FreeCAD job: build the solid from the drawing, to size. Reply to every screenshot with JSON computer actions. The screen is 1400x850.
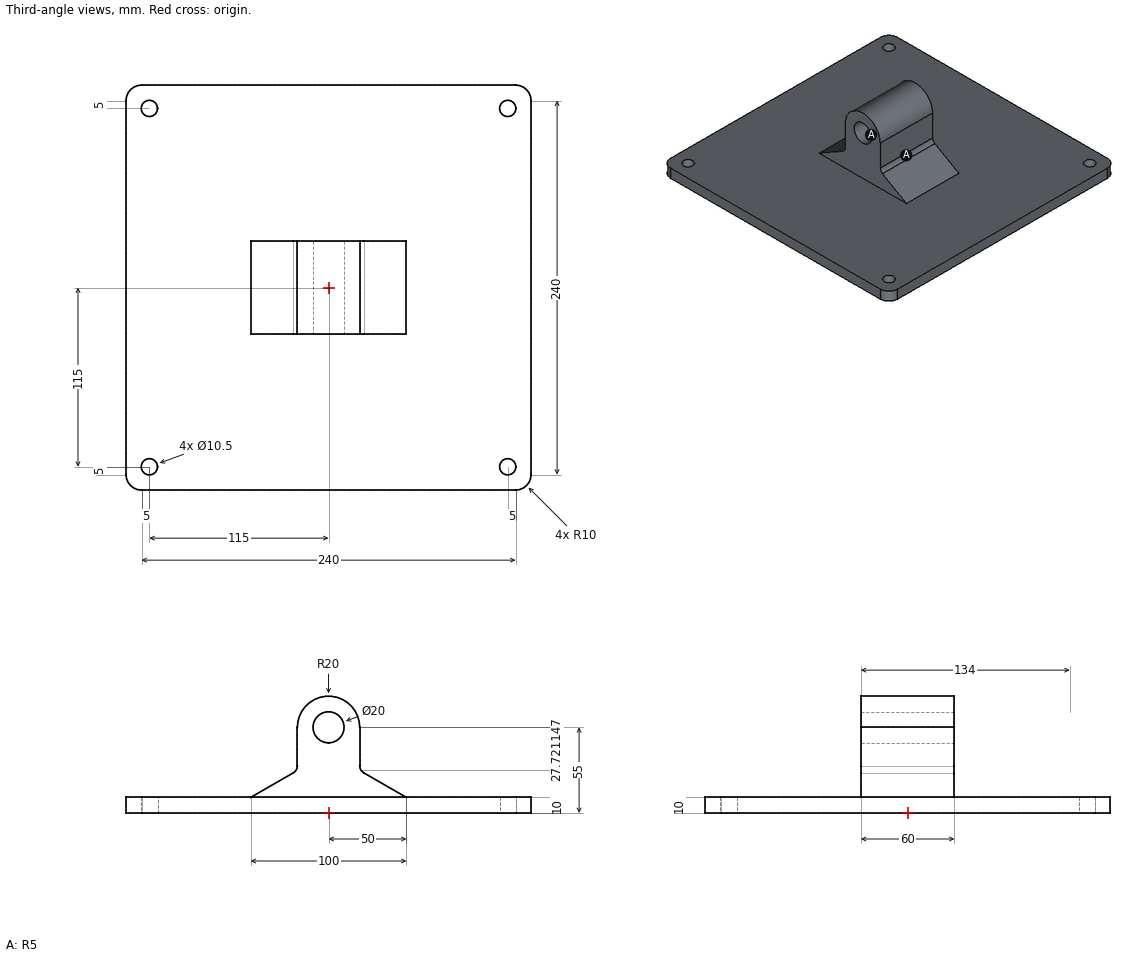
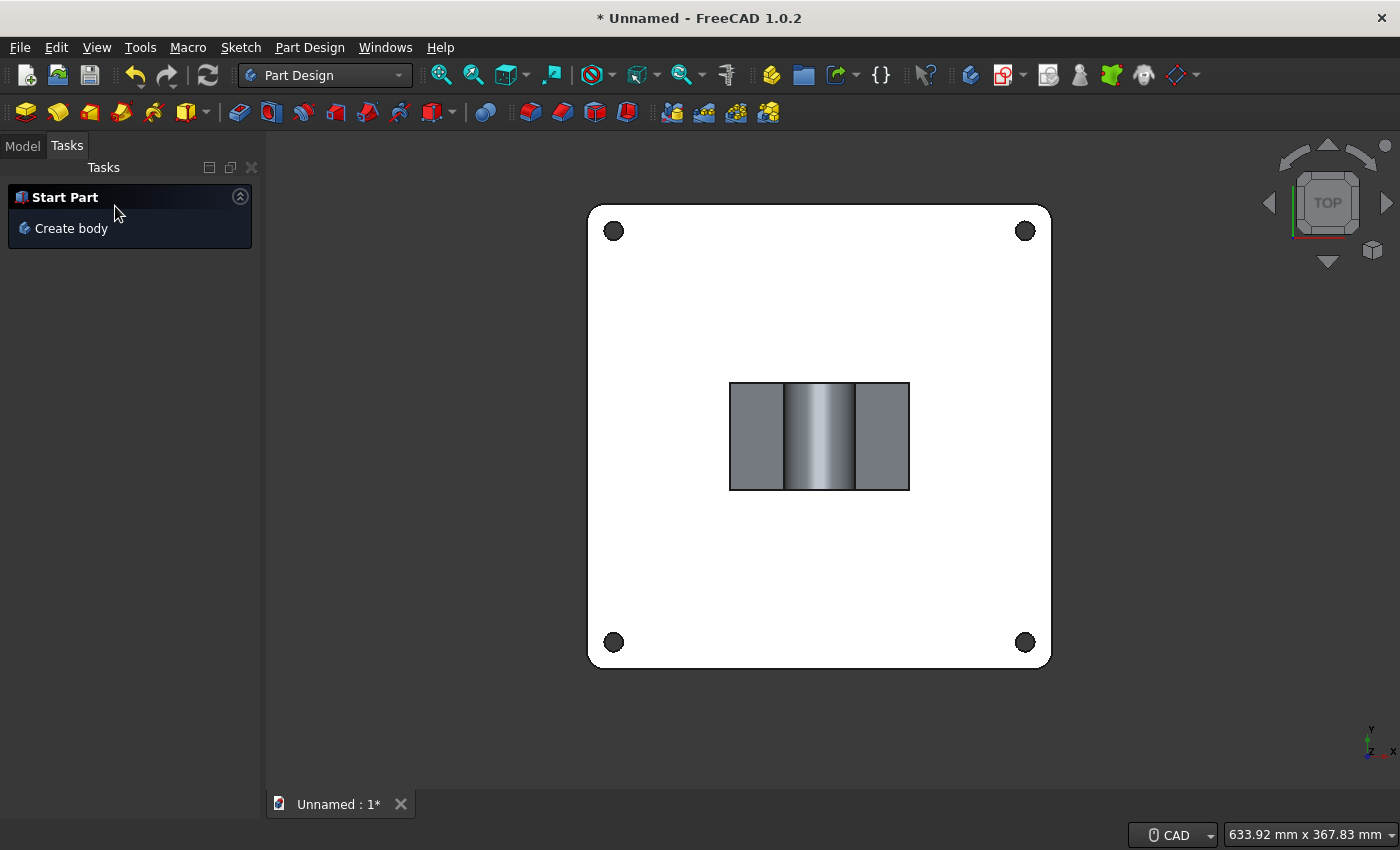
{"action": "key", "text": "1"}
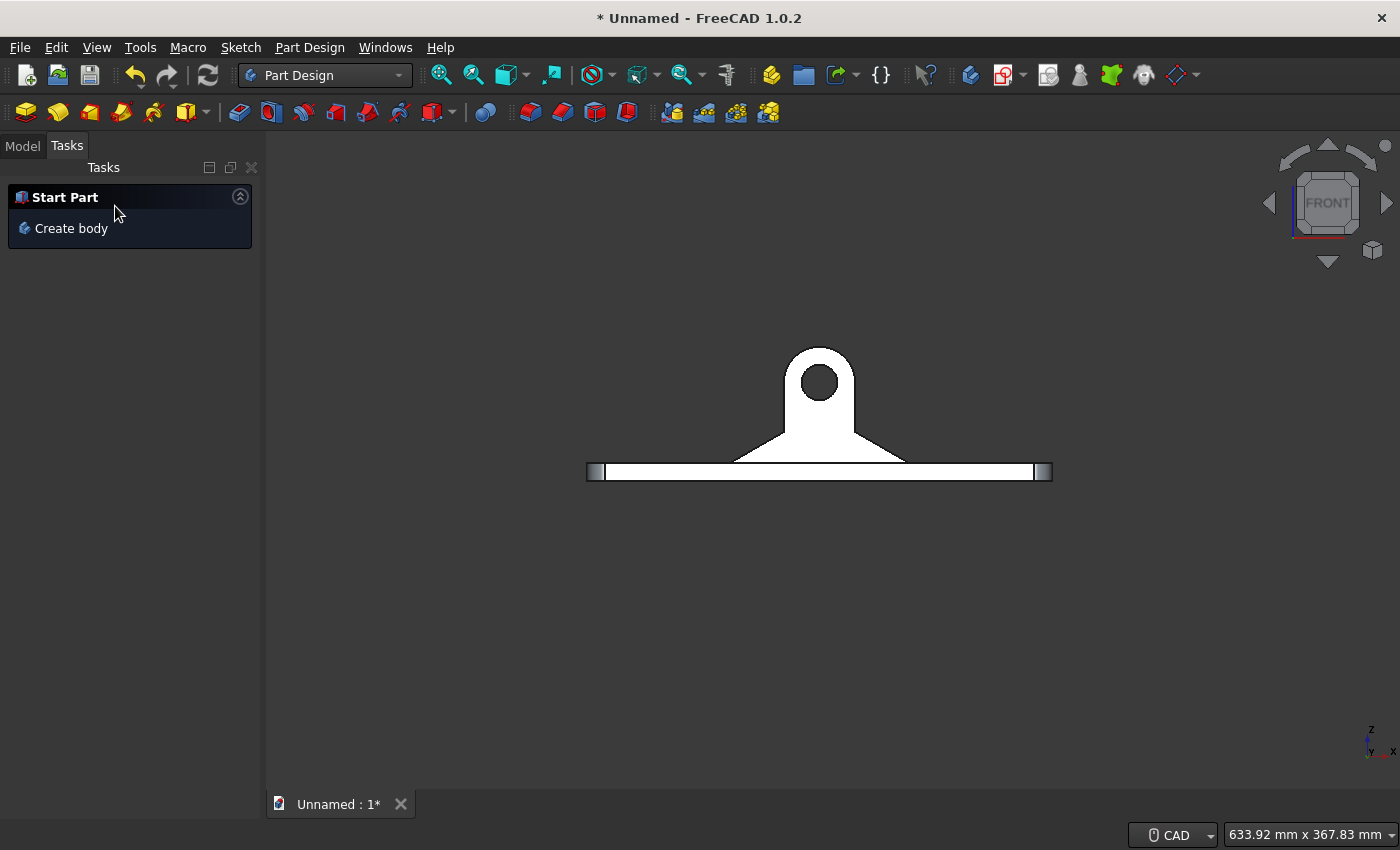
{"action": "left_click", "coordinate": [442, 76]}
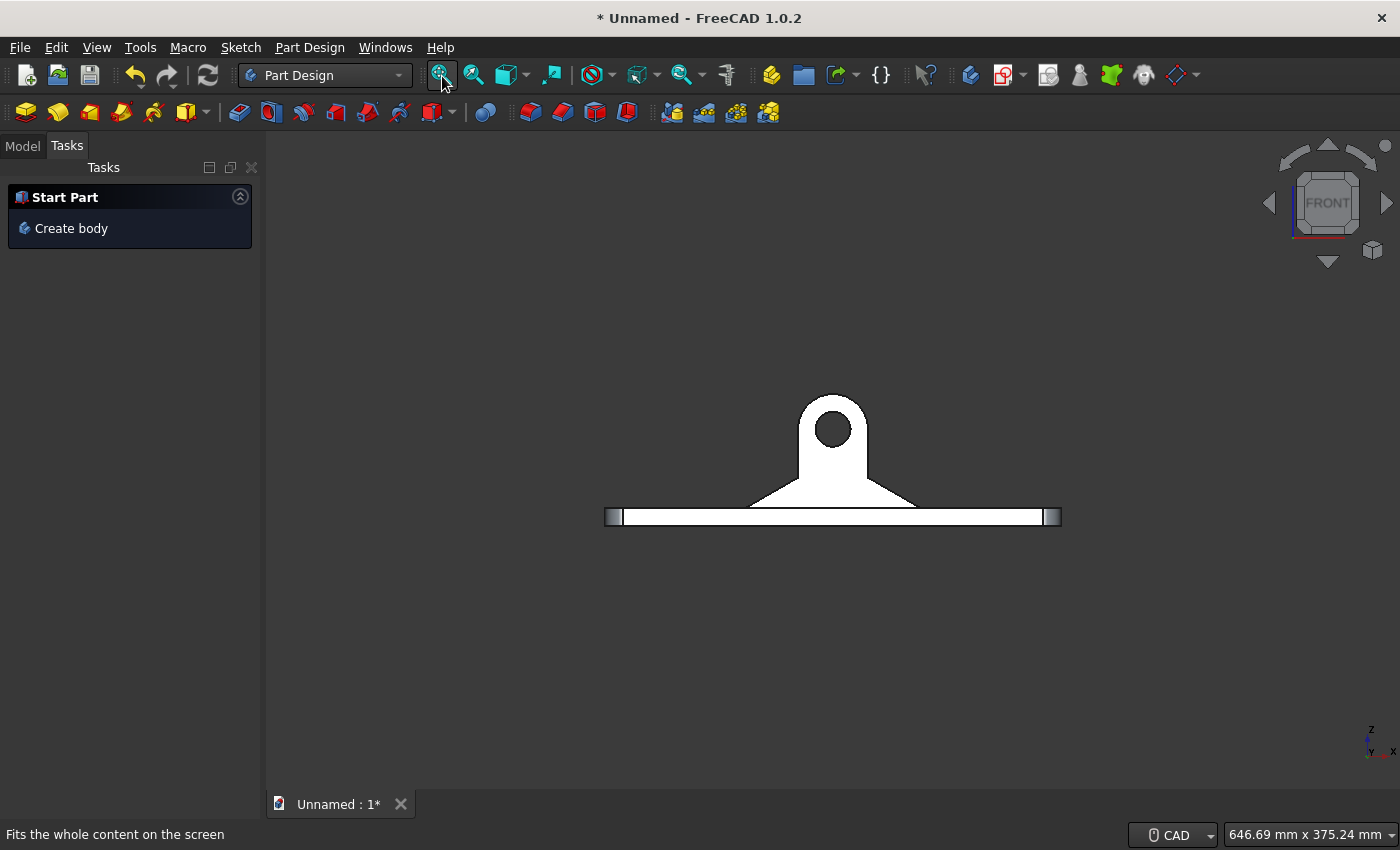
{"action": "key", "text": "3"}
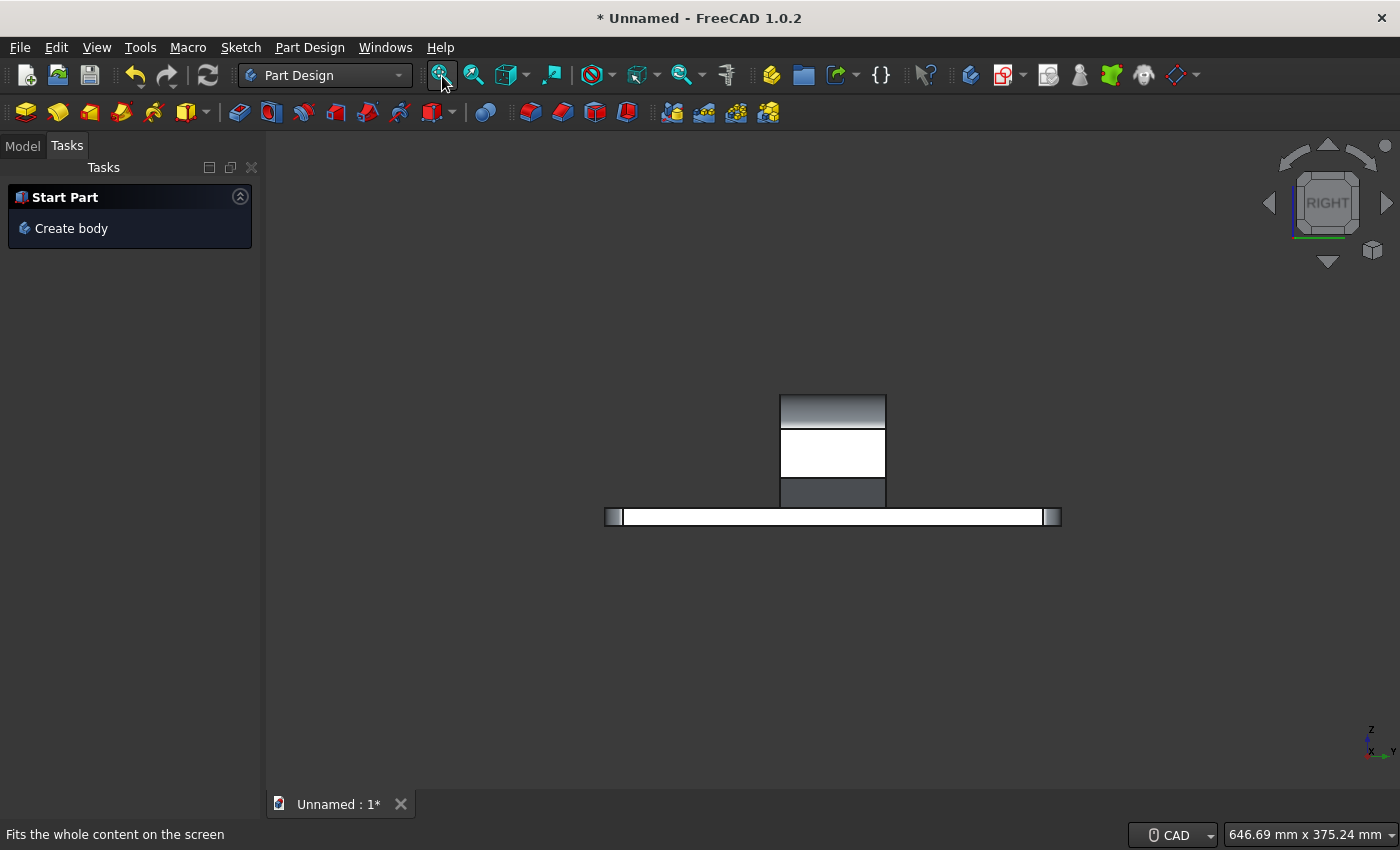
{"action": "left_click", "coordinate": [442, 76]}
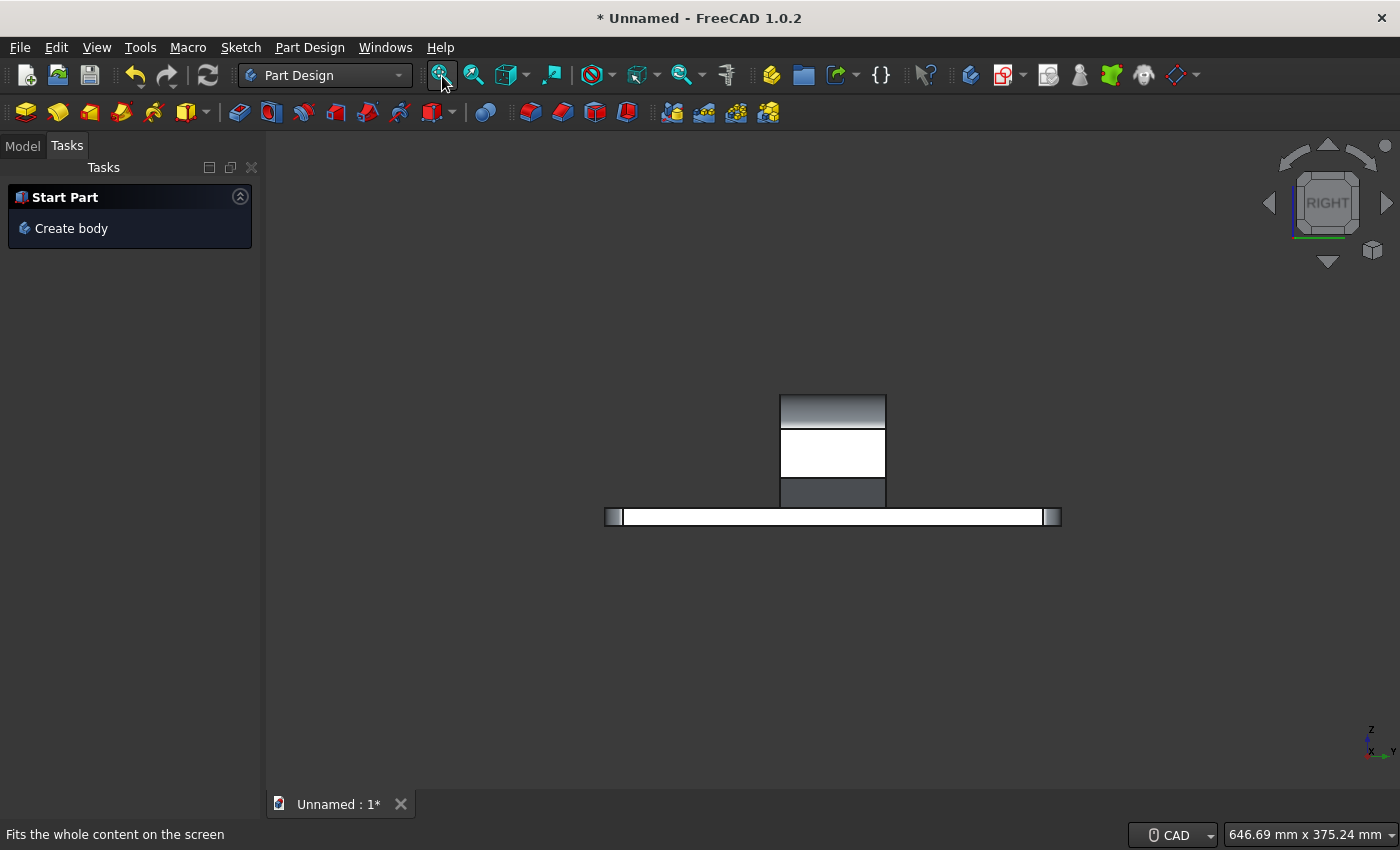
{"action": "key", "text": "5"}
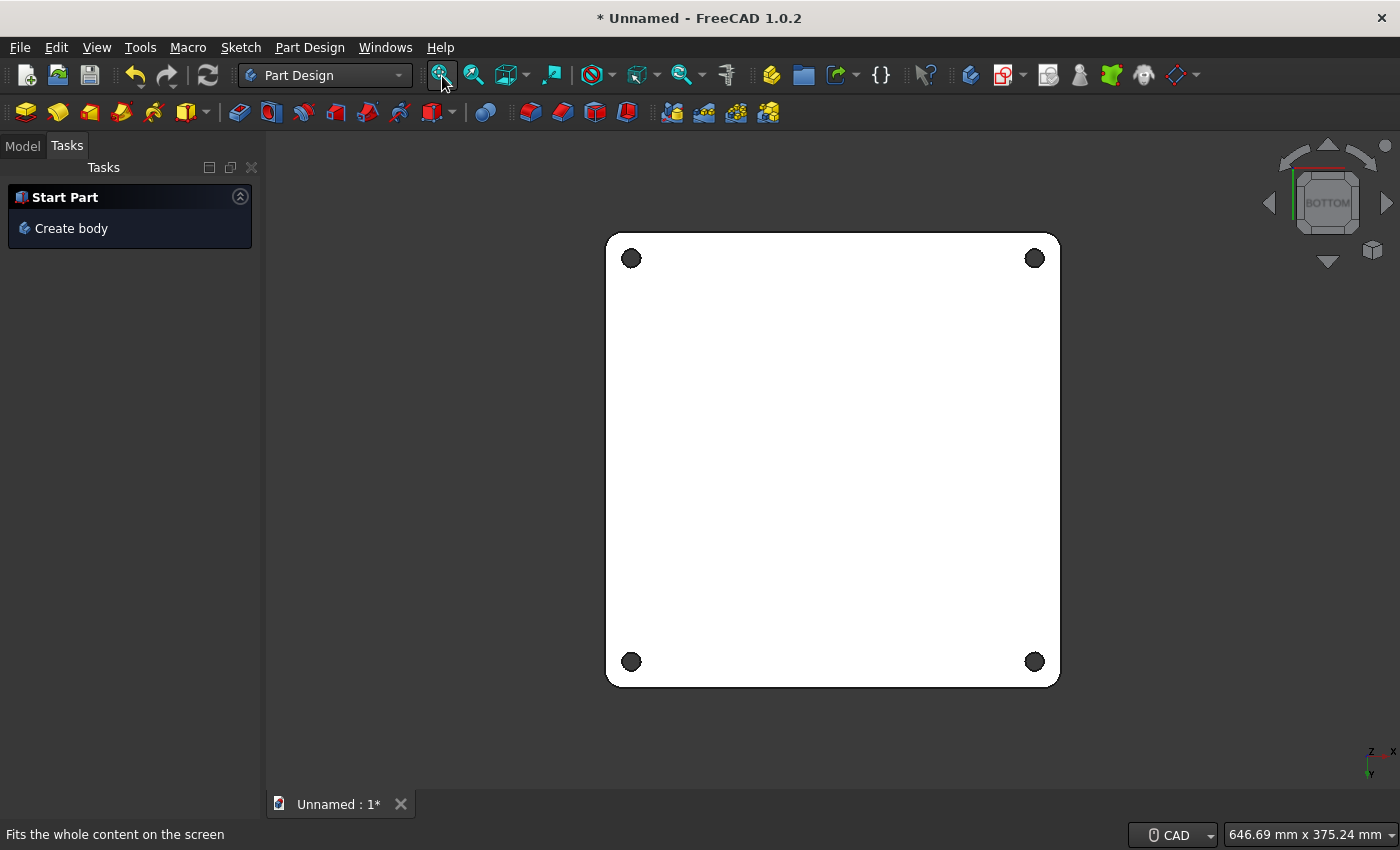
{"action": "key", "text": "4"}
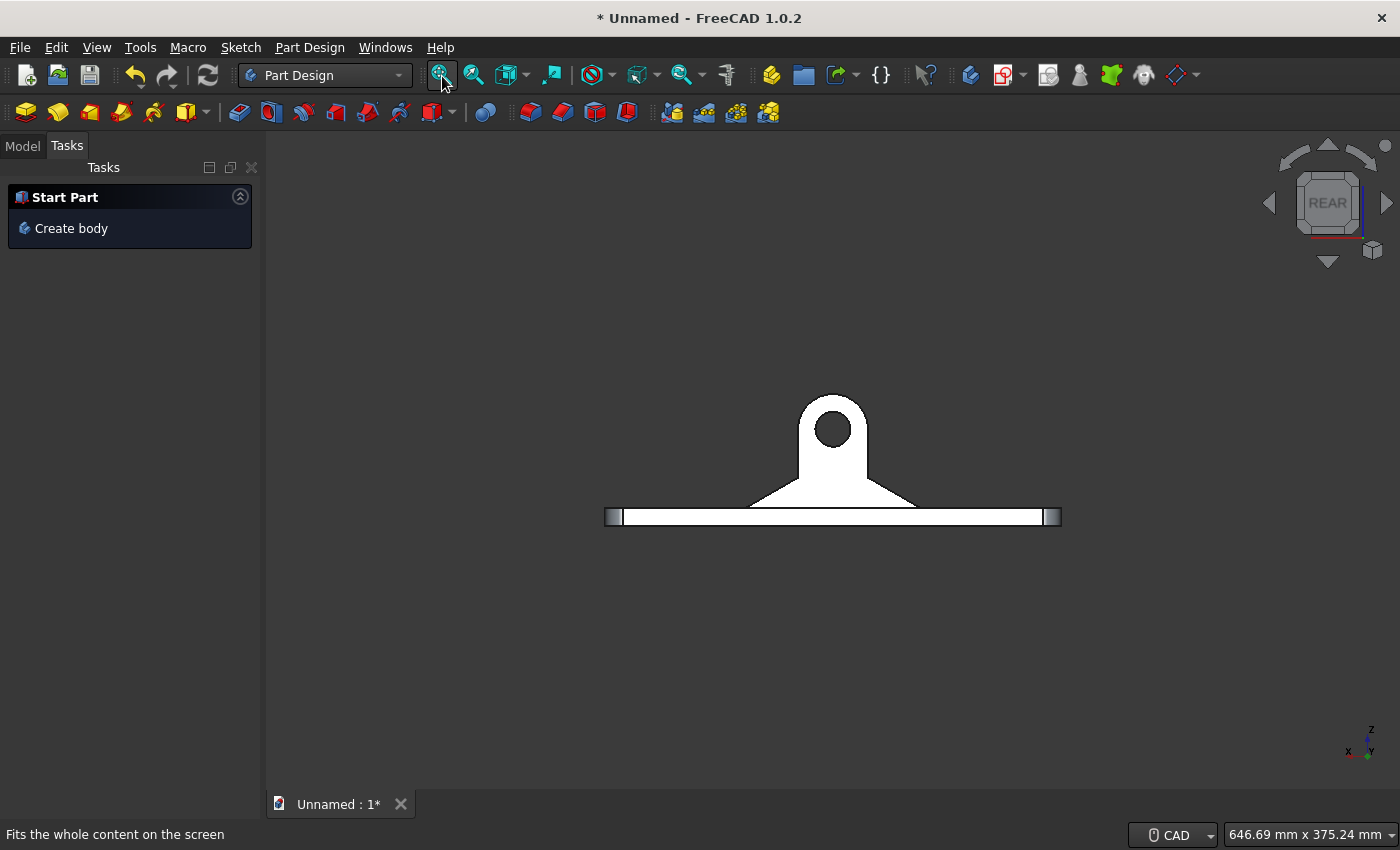
{"action": "left_click", "coordinate": [442, 76]}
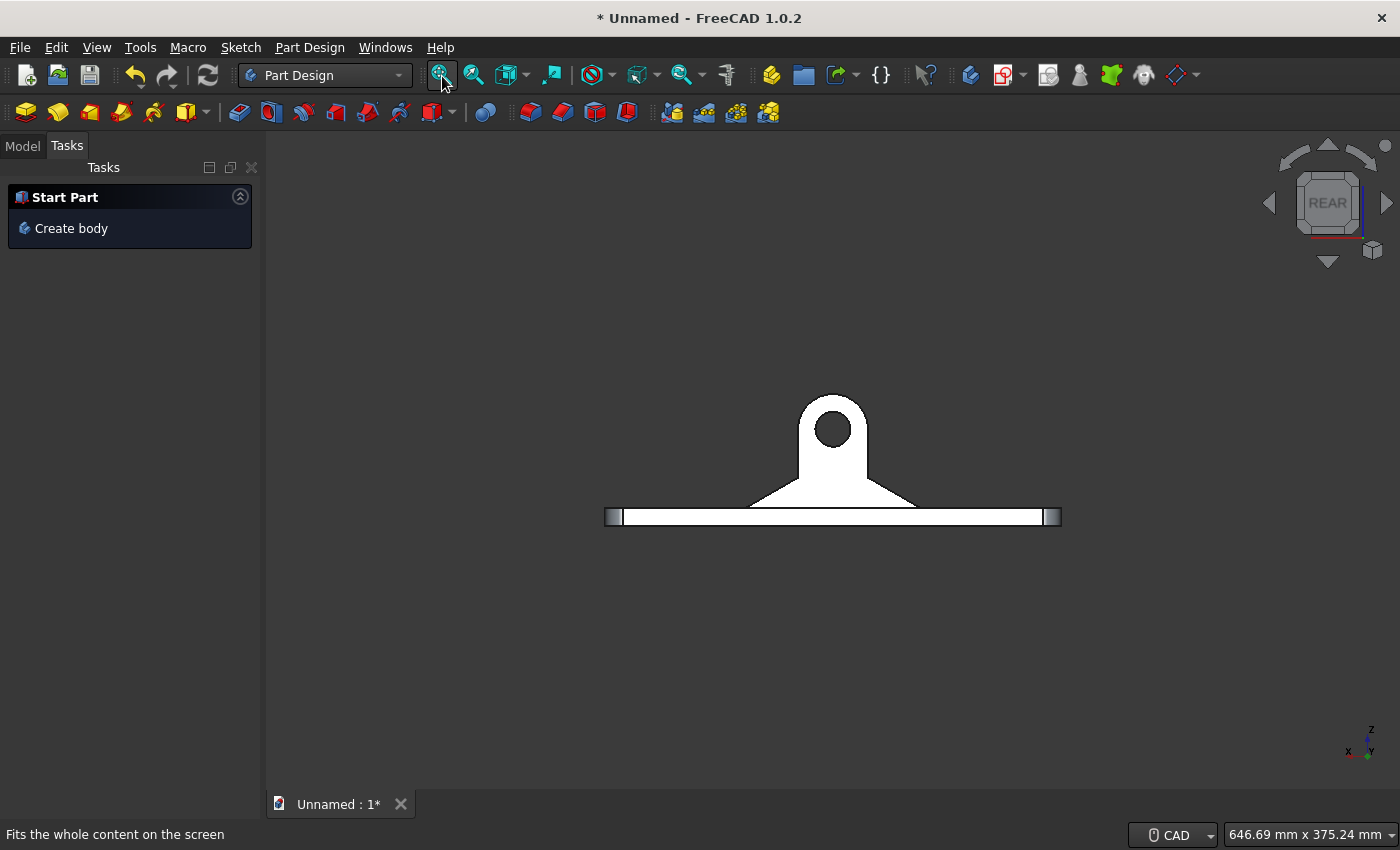
{"action": "key", "text": "6"}